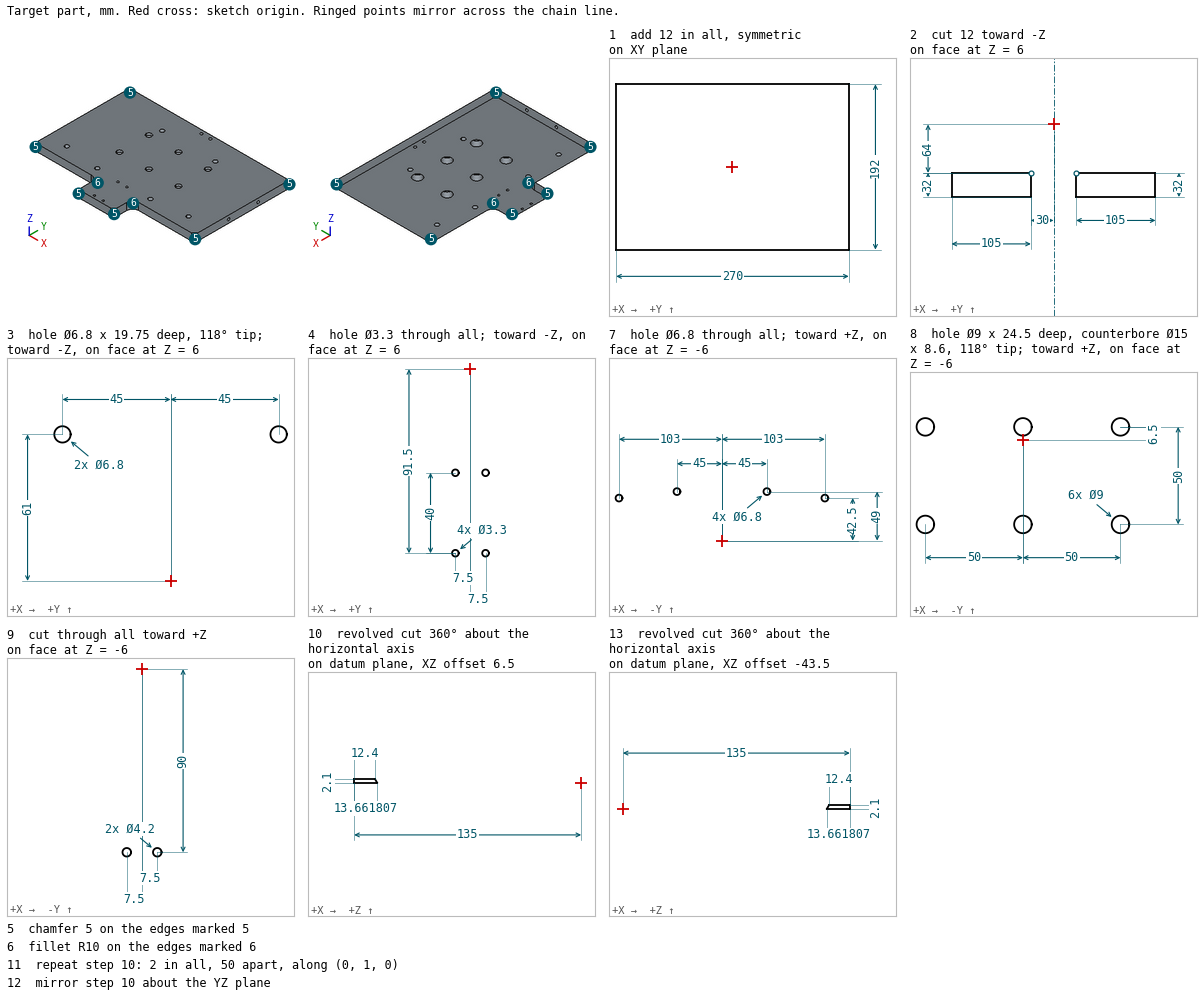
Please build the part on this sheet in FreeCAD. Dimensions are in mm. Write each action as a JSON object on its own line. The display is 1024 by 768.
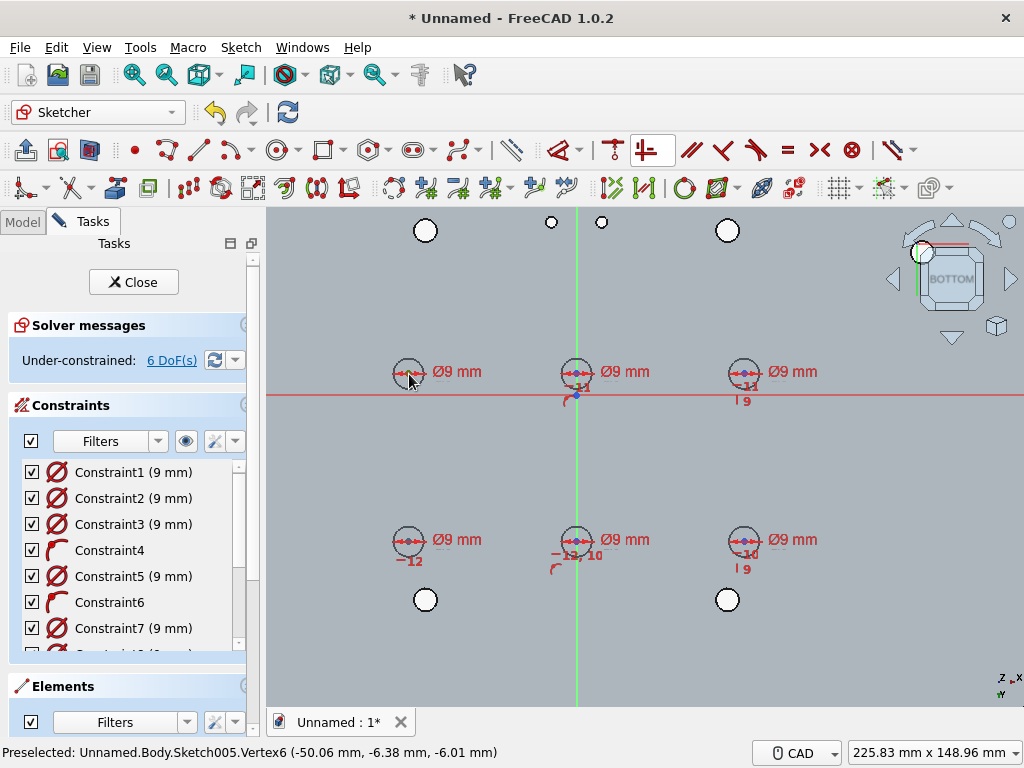
{"action": "left_click", "coordinate": [670, 150]}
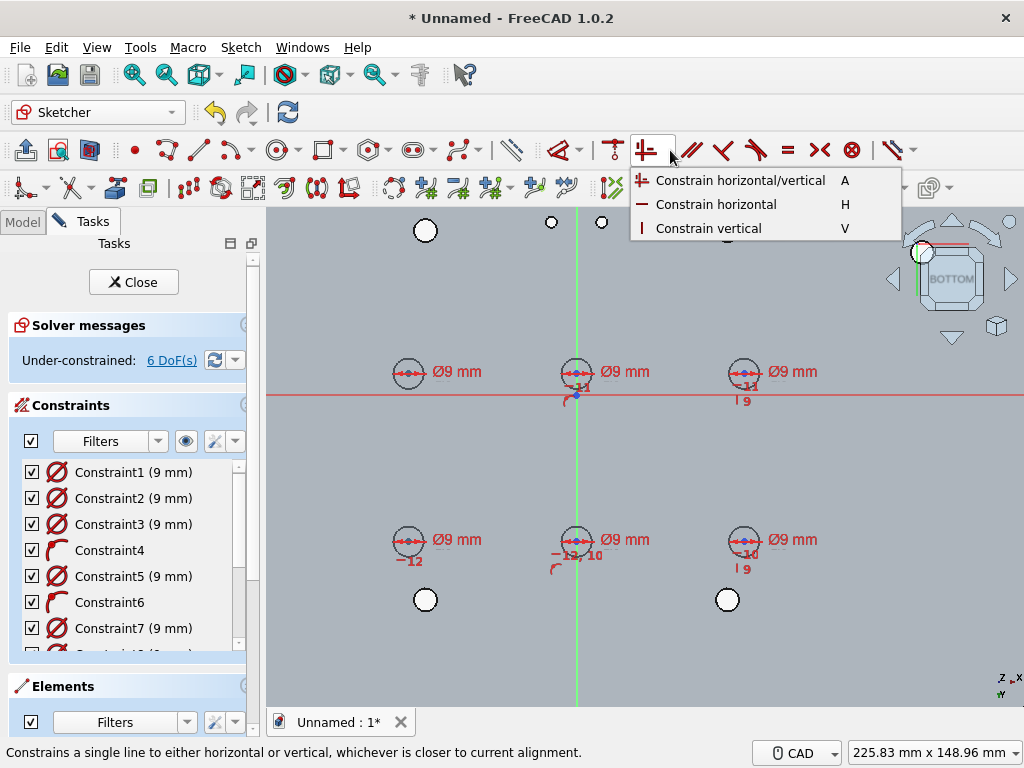
{"action": "left_click", "coordinate": [766, 228]}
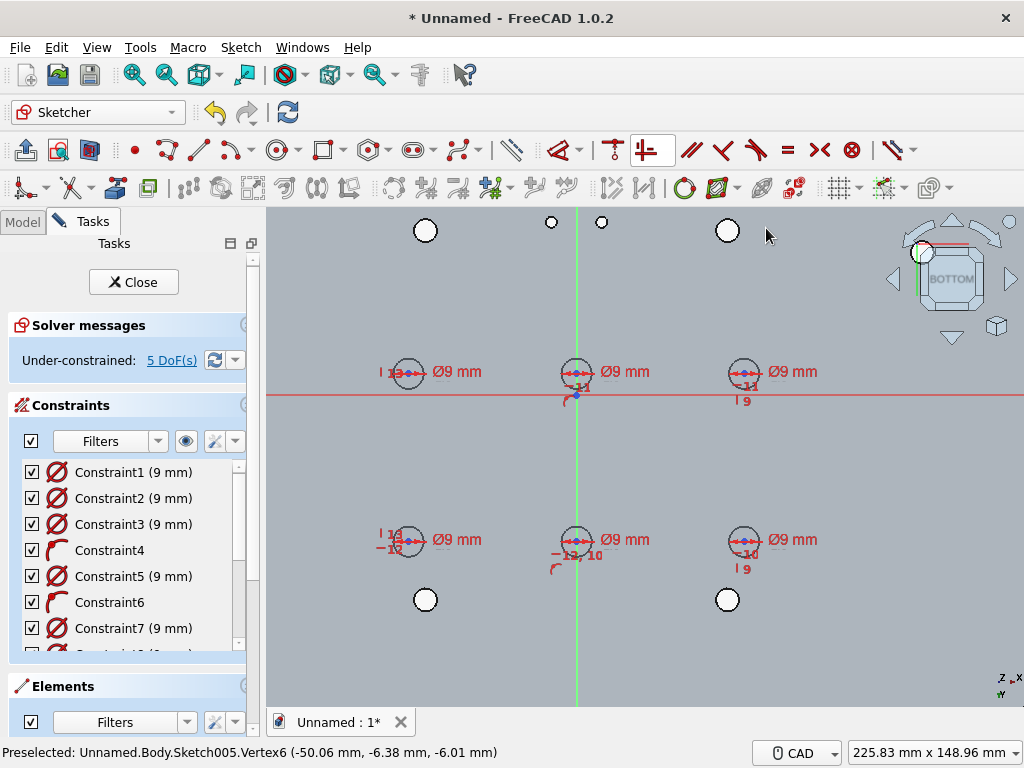
{"action": "left_click", "coordinate": [577, 374]}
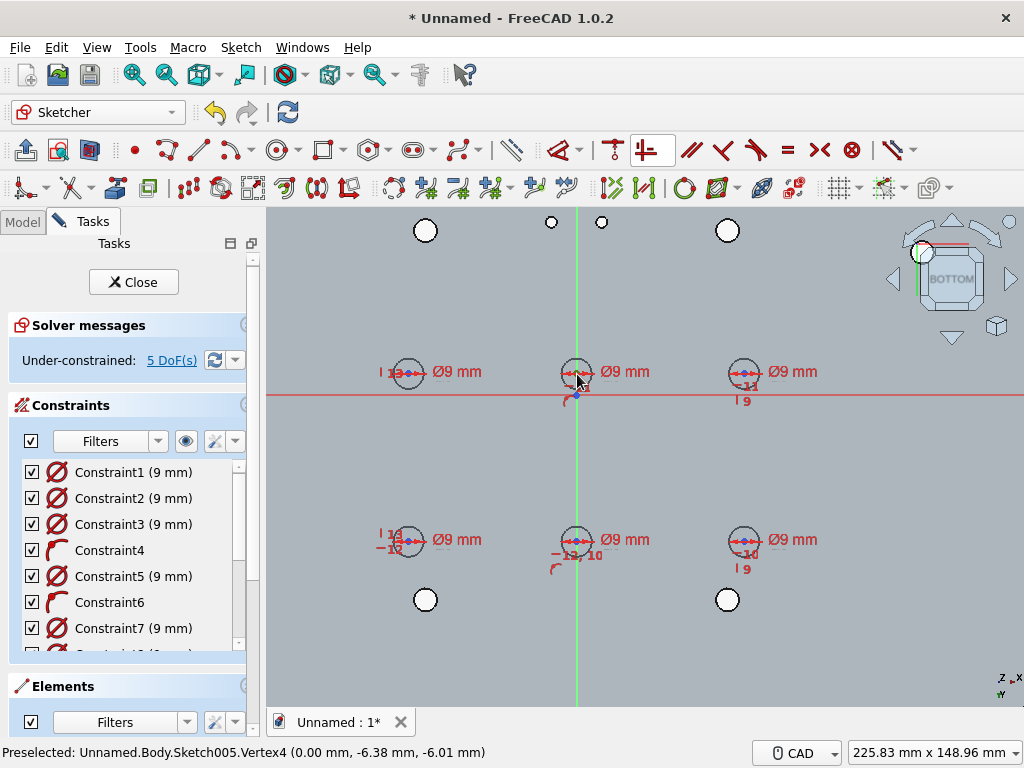
{"action": "left_click", "coordinate": [409, 374]}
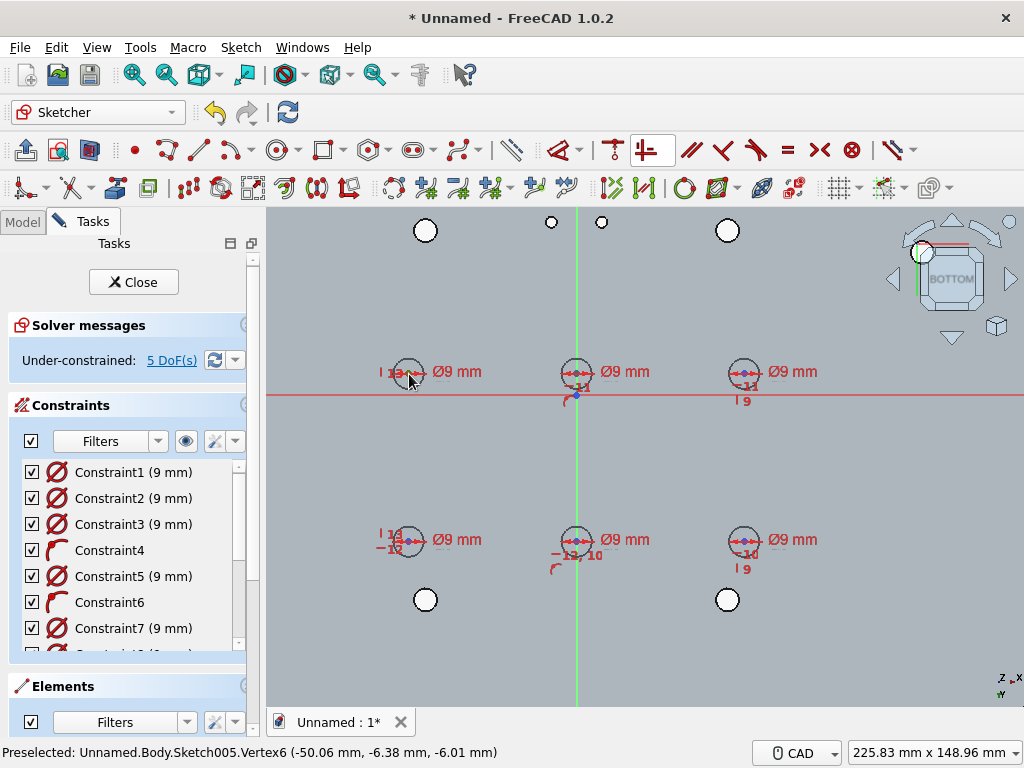
{"action": "key", "text": "h"}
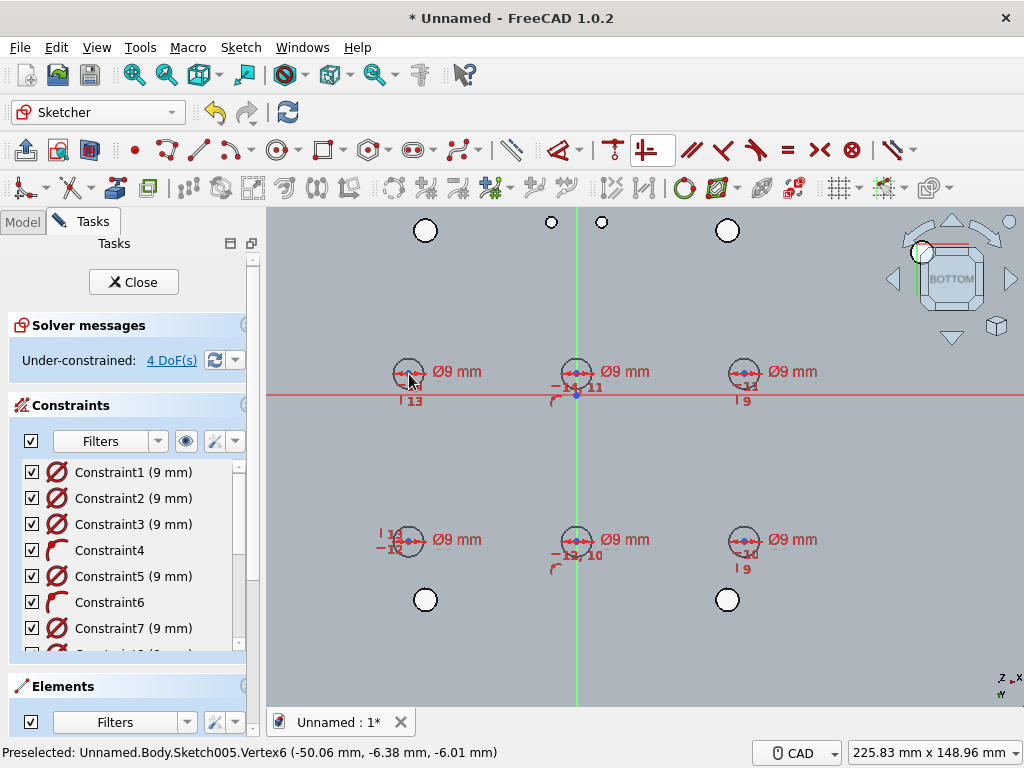
{"action": "key", "text": "d"}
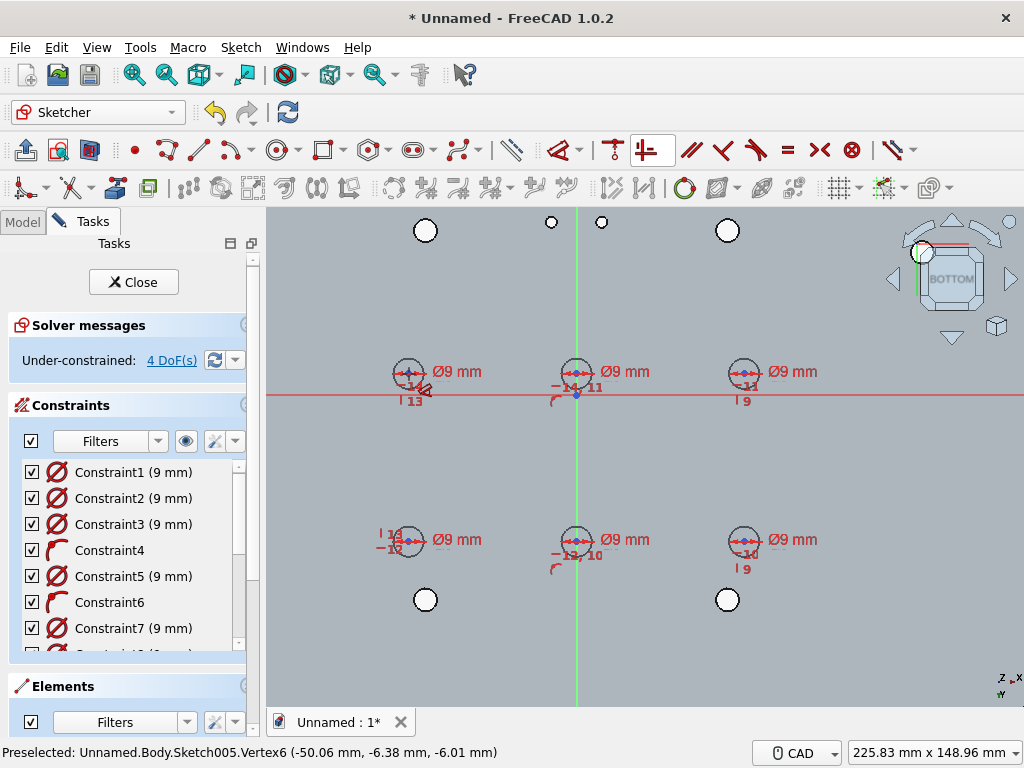
{"action": "left_click", "coordinate": [744, 542]}
{"action": "left_click", "coordinate": [660, 576]}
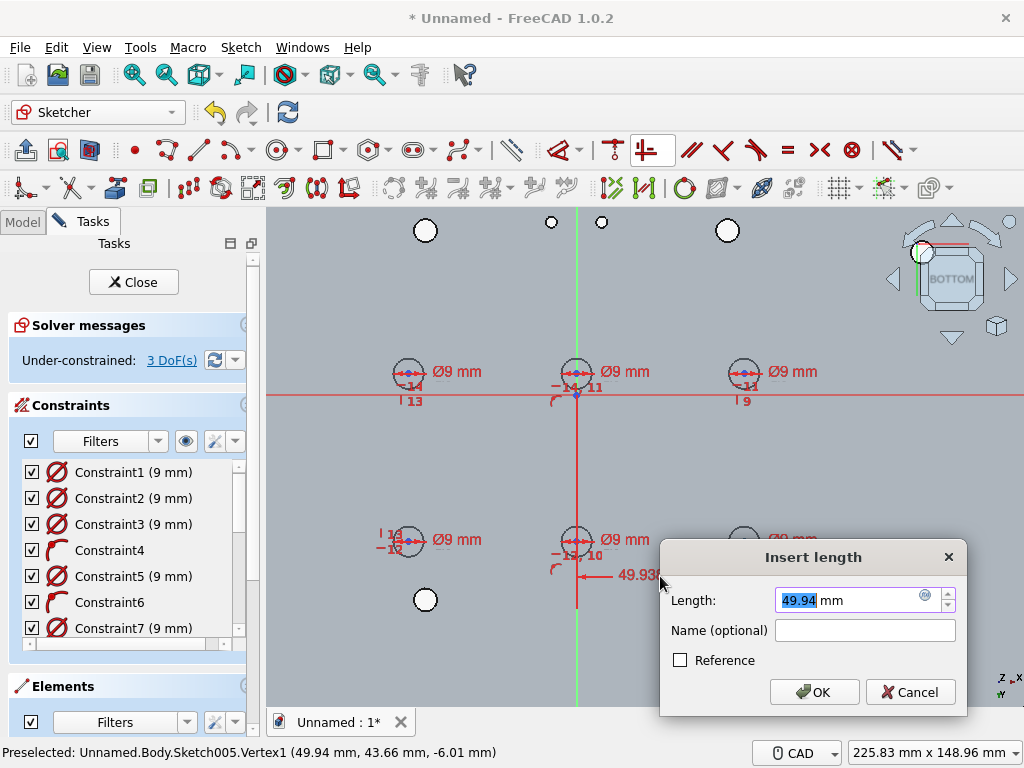
{"action": "type", "text": "50"}
{"action": "key", "text": "Return"}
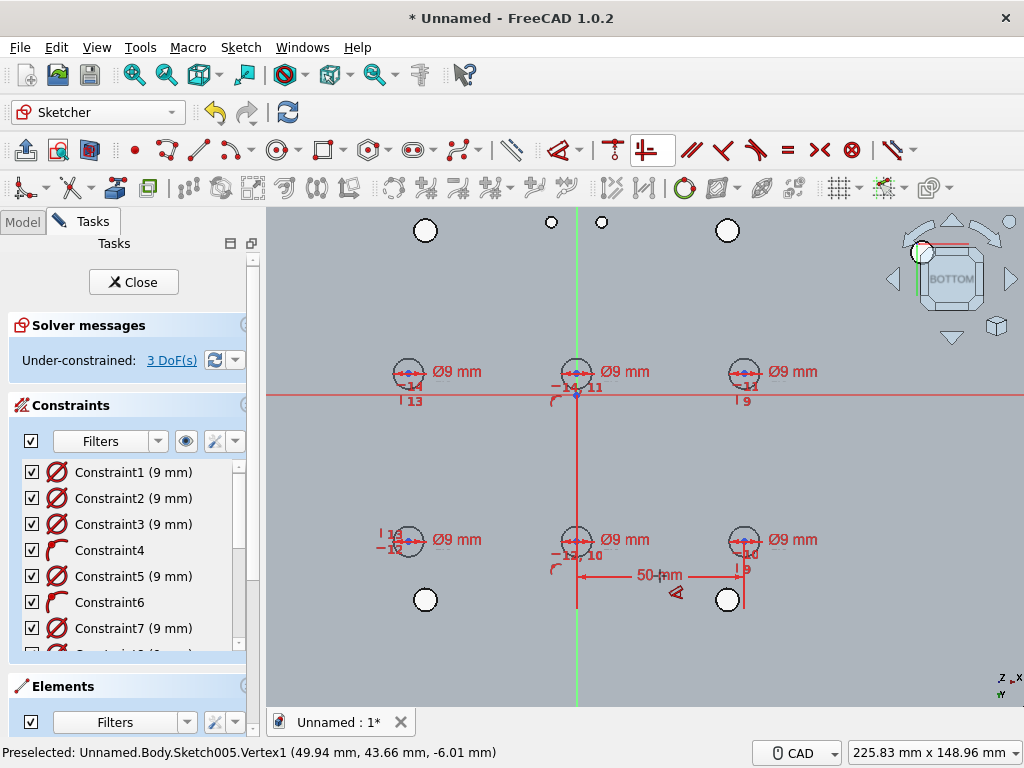
{"action": "left_click", "coordinate": [409, 542]}
{"action": "left_click", "coordinate": [493, 576]}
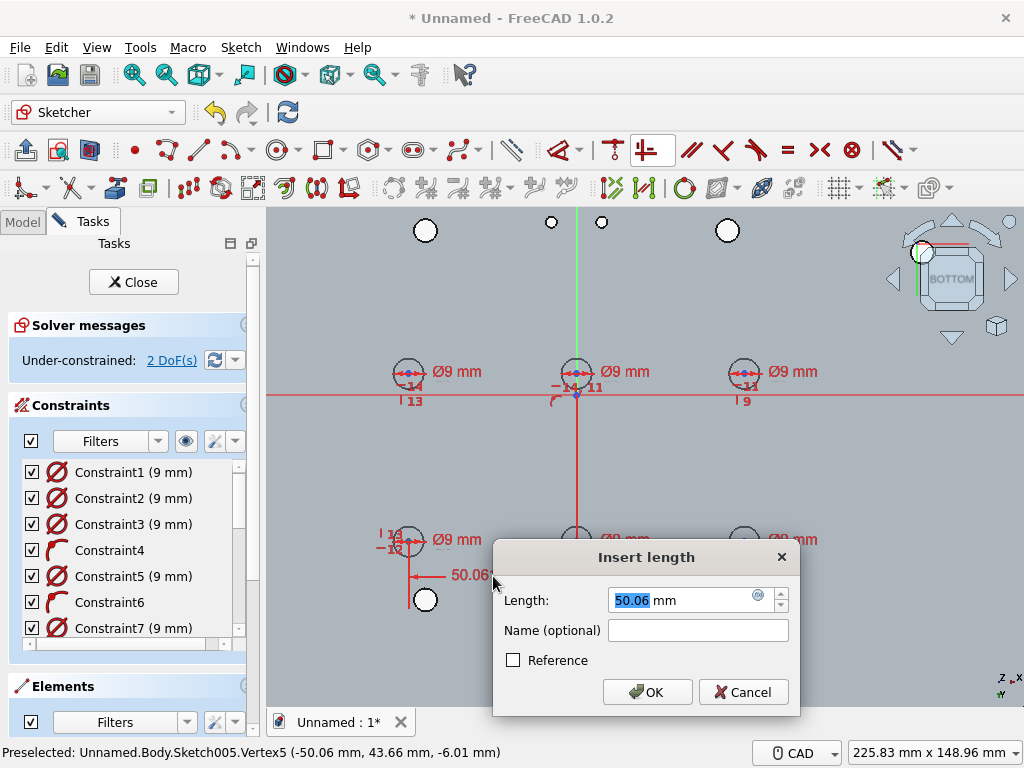
{"action": "type", "text": "50"}
{"action": "key", "text": "Return"}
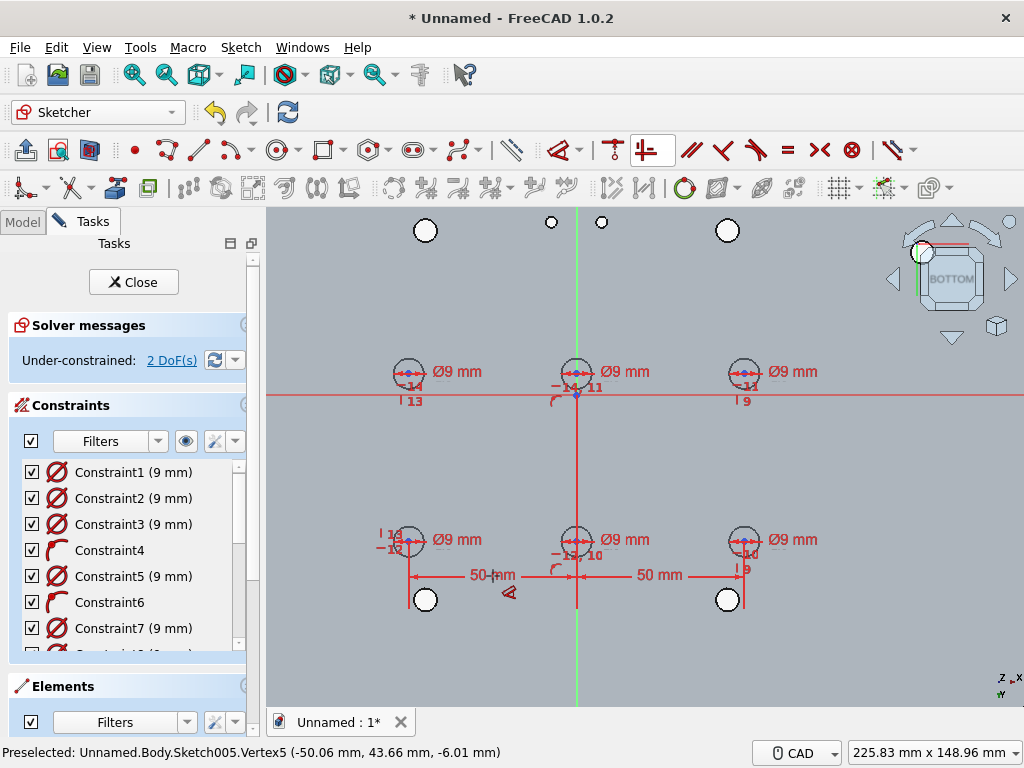
{"action": "scroll", "coordinate": [744, 374], "scroll_direction": "up", "scroll_amount": 3}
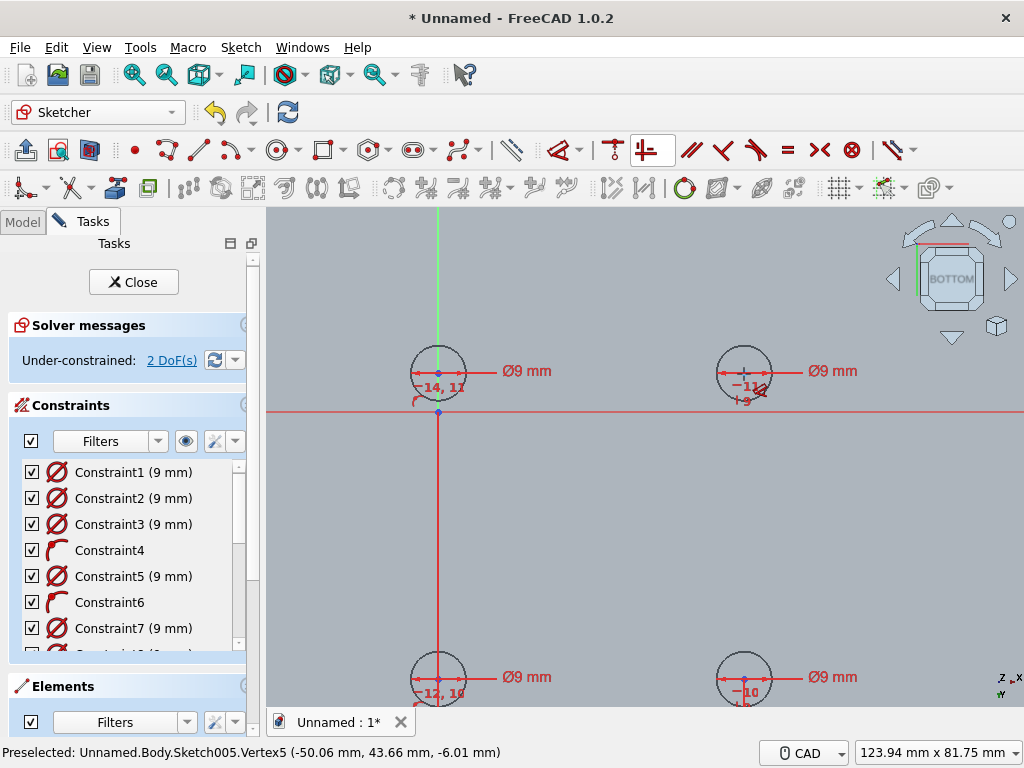
{"action": "left_click", "coordinate": [744, 373]}
{"action": "left_click", "coordinate": [802, 393]}